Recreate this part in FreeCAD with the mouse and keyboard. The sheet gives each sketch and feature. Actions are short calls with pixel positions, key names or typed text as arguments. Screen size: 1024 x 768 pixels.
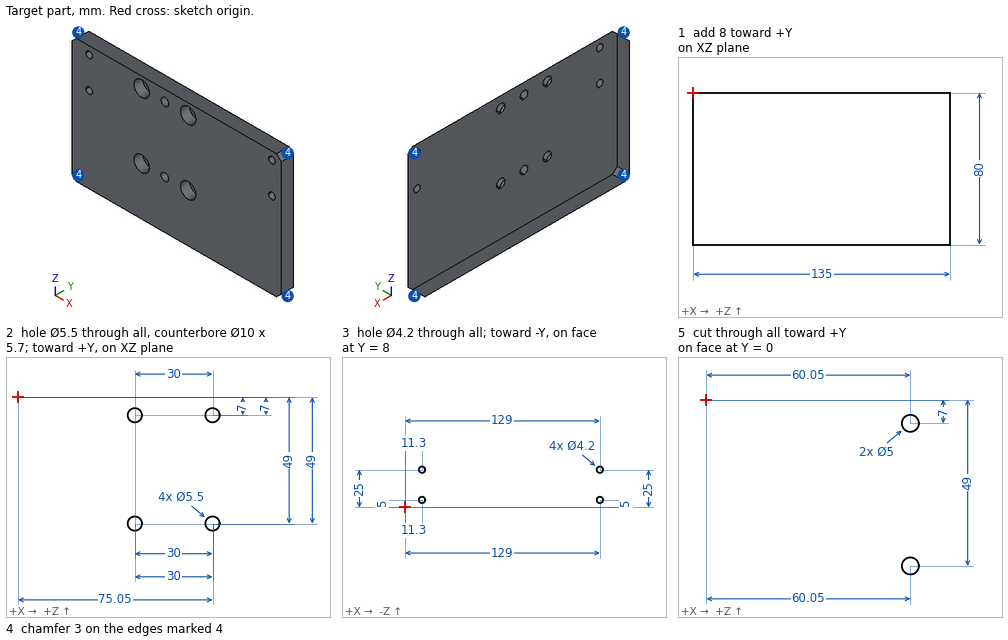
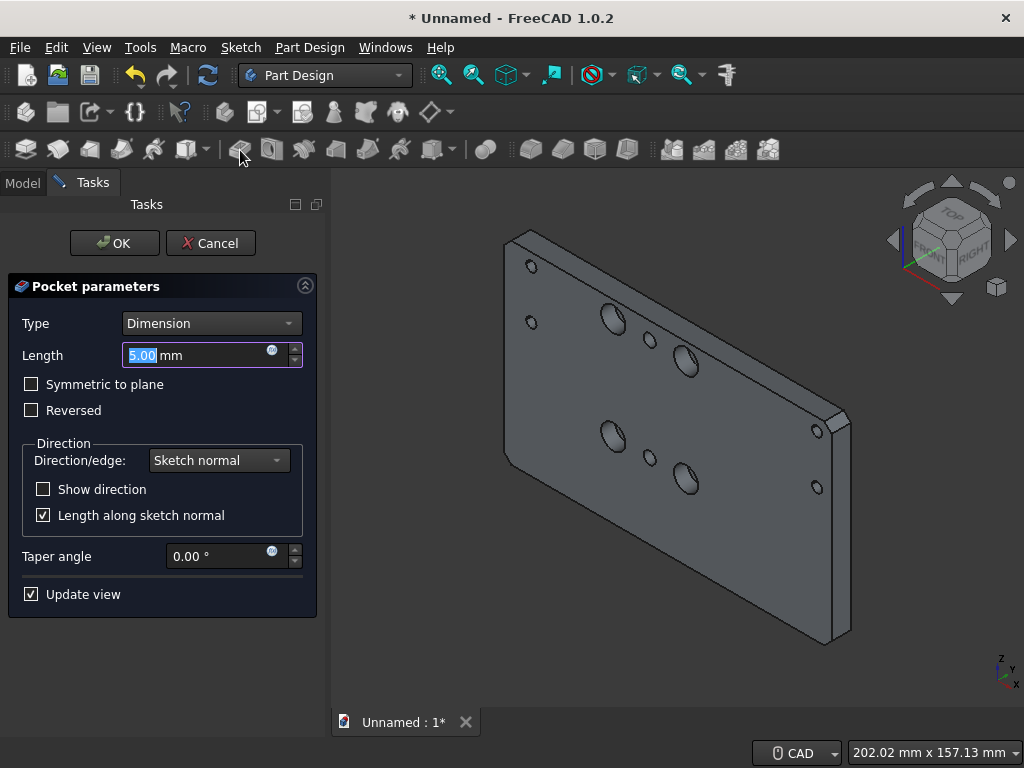
click(212, 324)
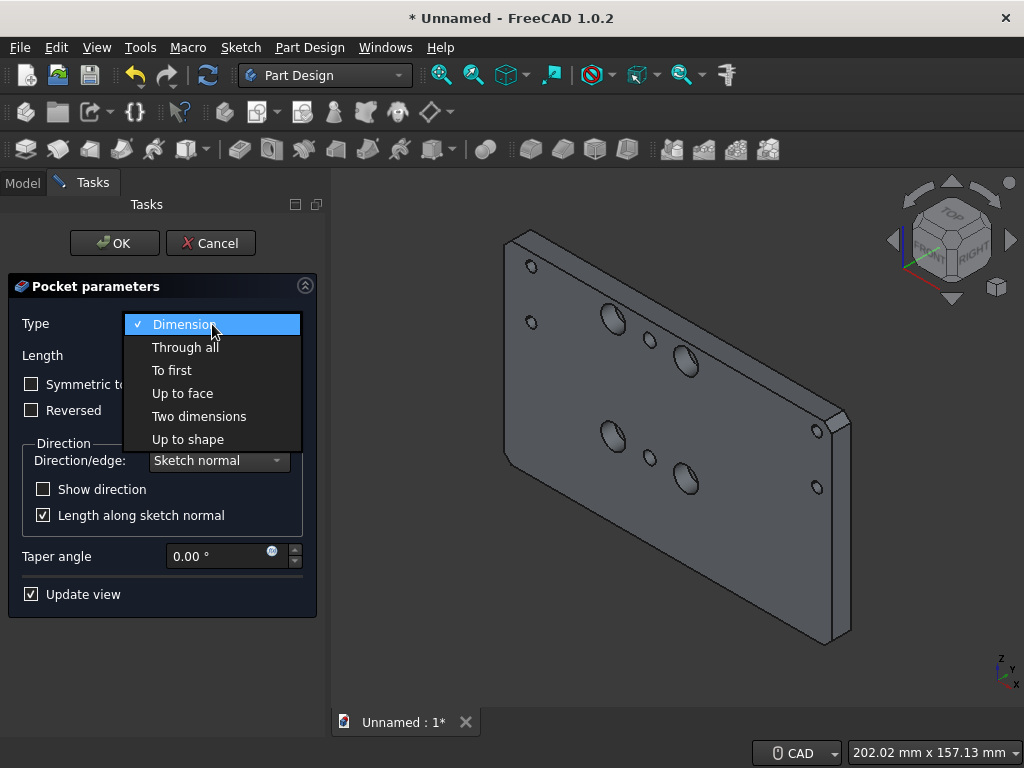
click(212, 348)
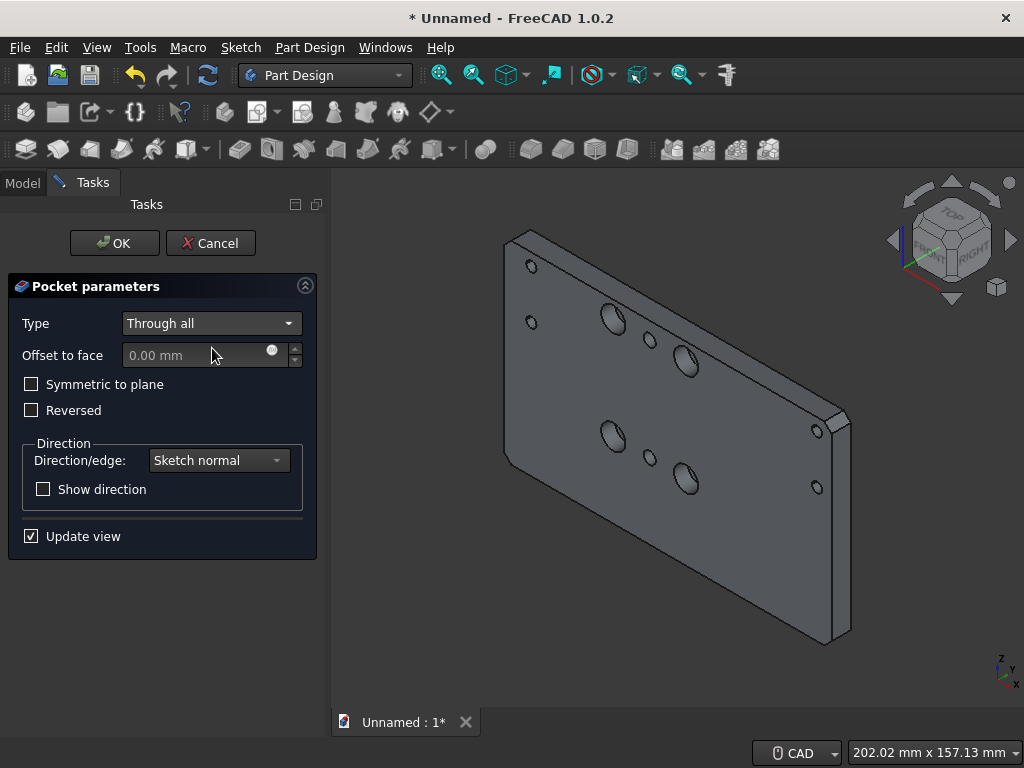
click(115, 243)